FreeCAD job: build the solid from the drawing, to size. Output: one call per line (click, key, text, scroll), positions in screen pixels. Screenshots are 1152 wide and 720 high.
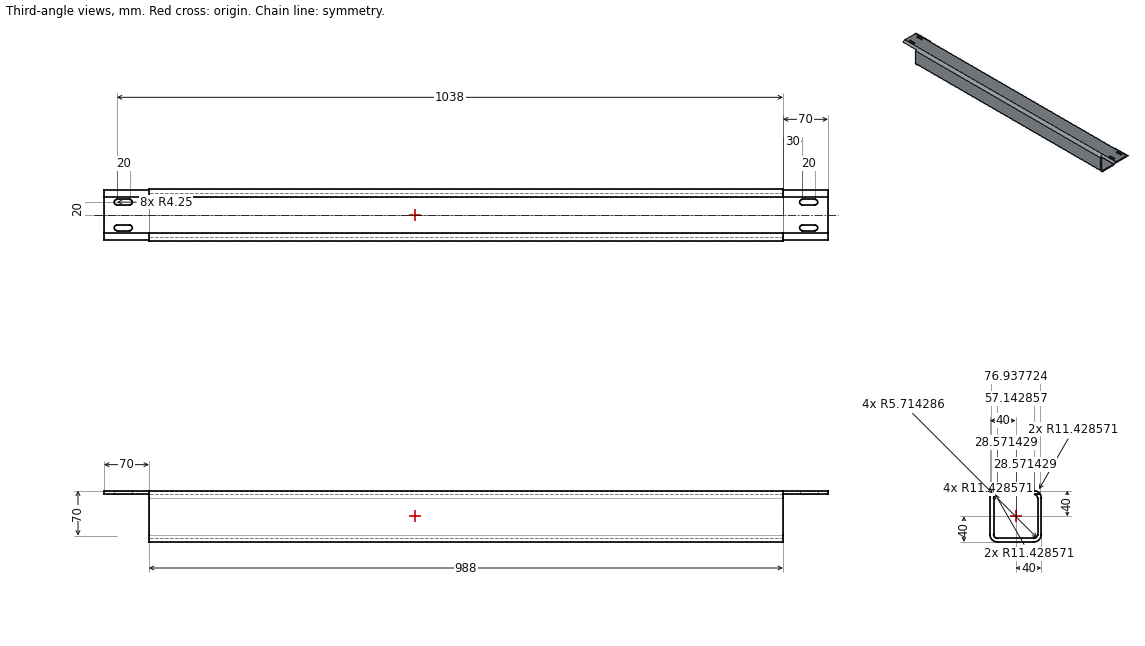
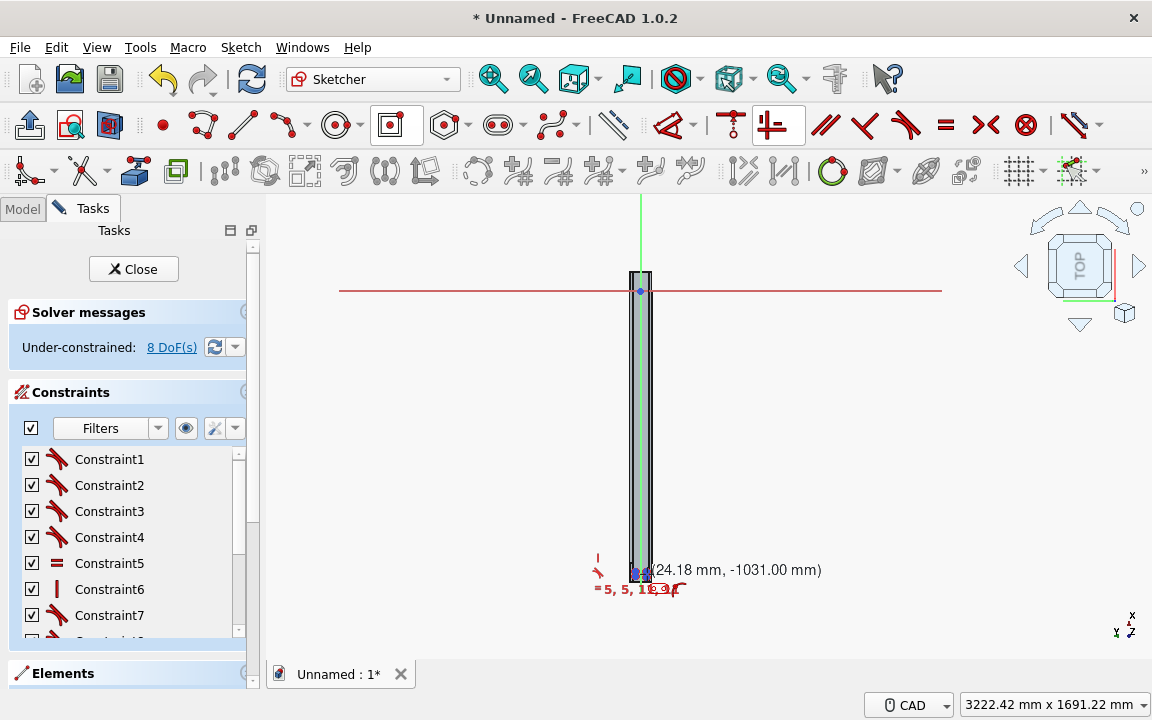
scroll(635, 283, up, 15)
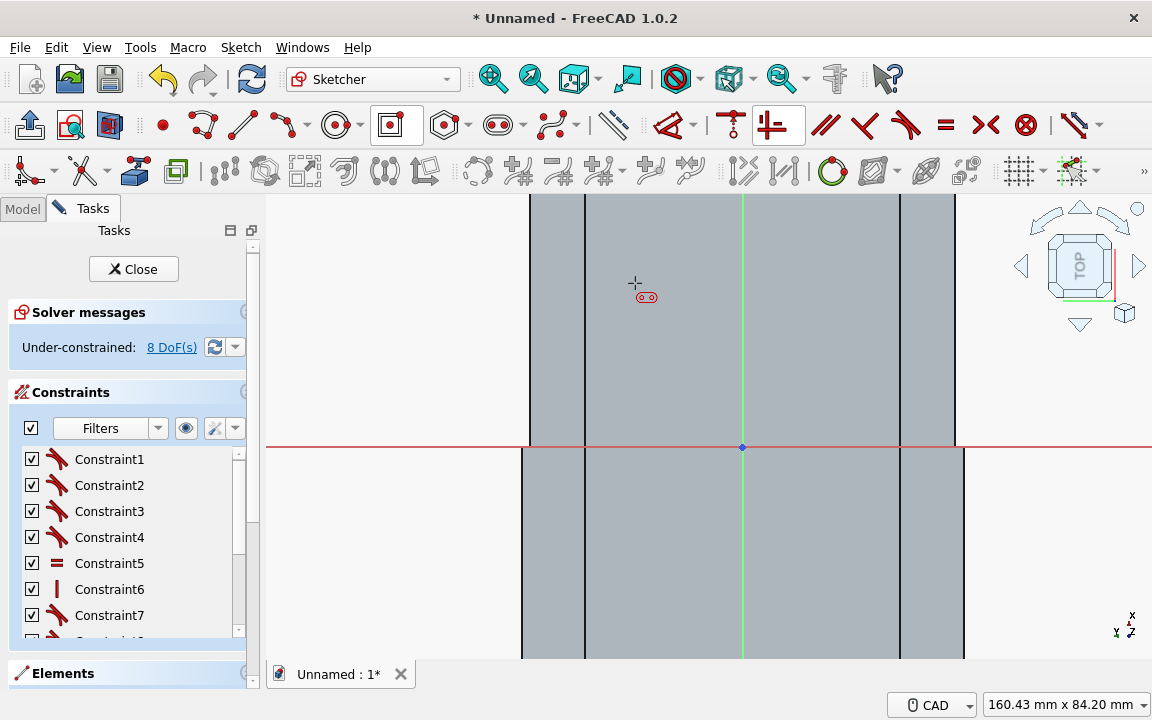
scroll(635, 282, down, 15)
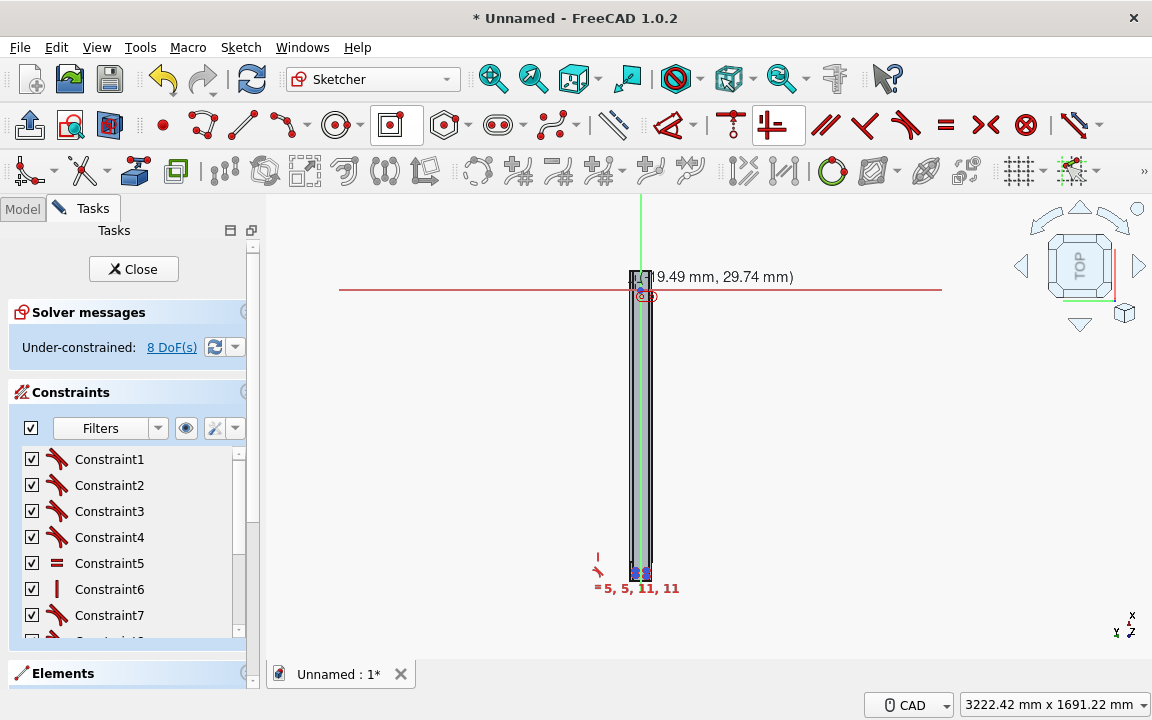
scroll(635, 282, up, 6)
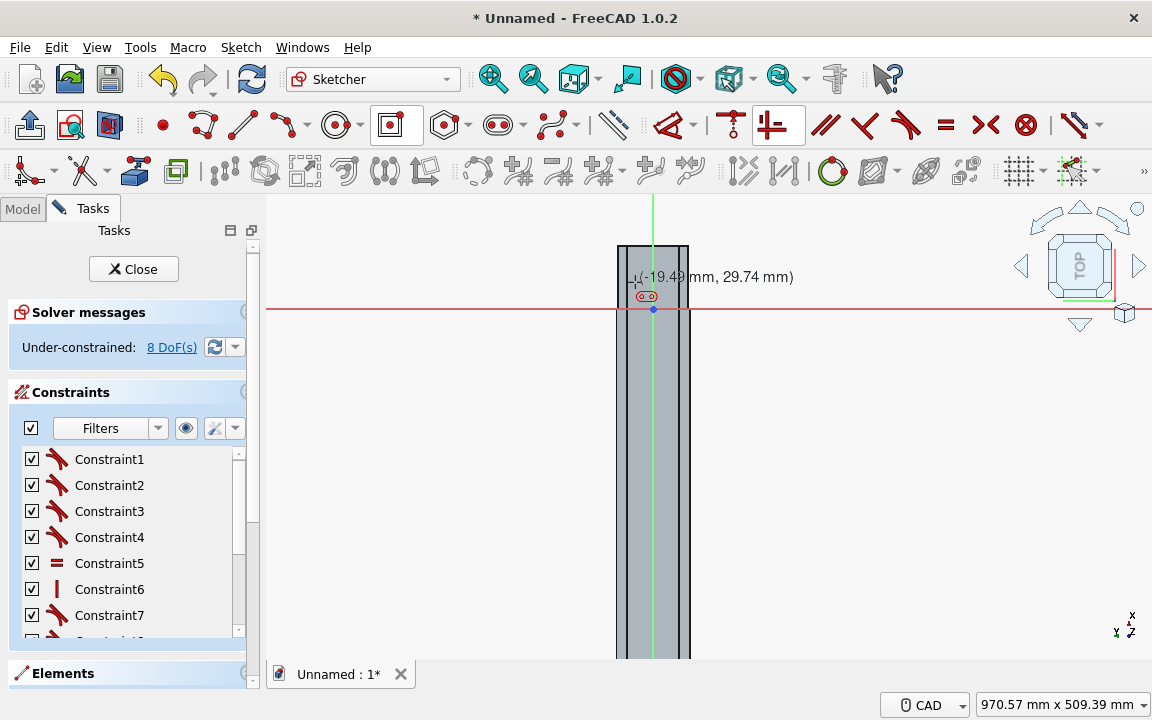
click(635, 282)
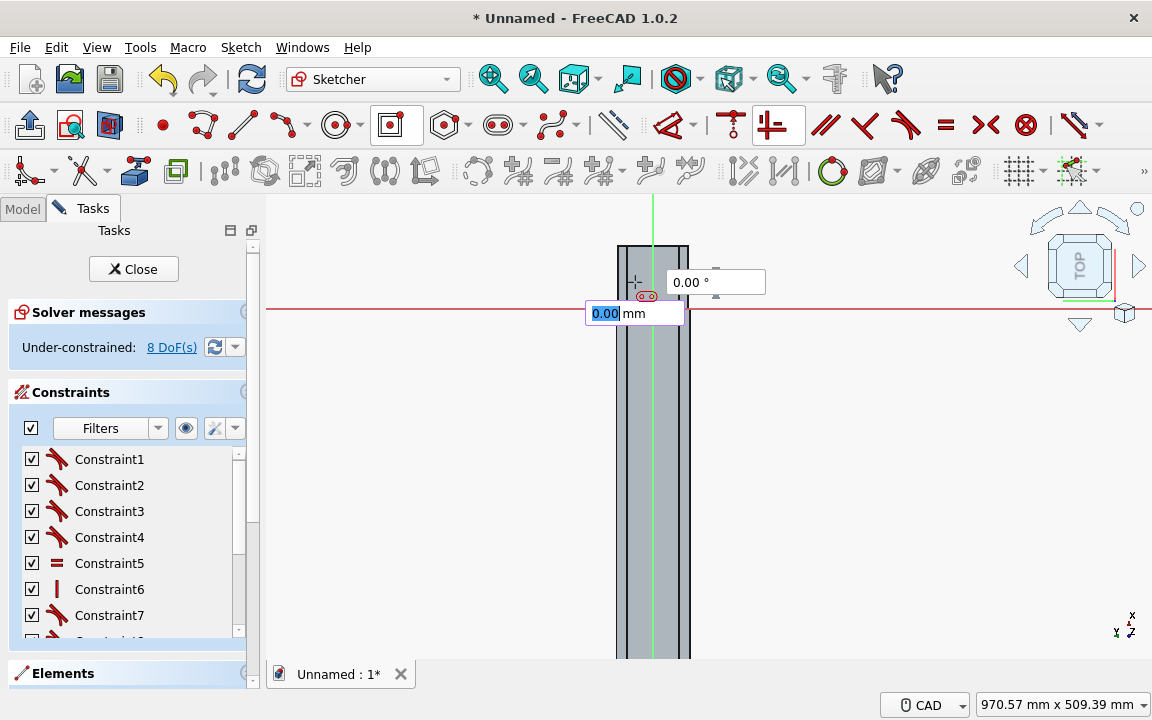
click(635, 264)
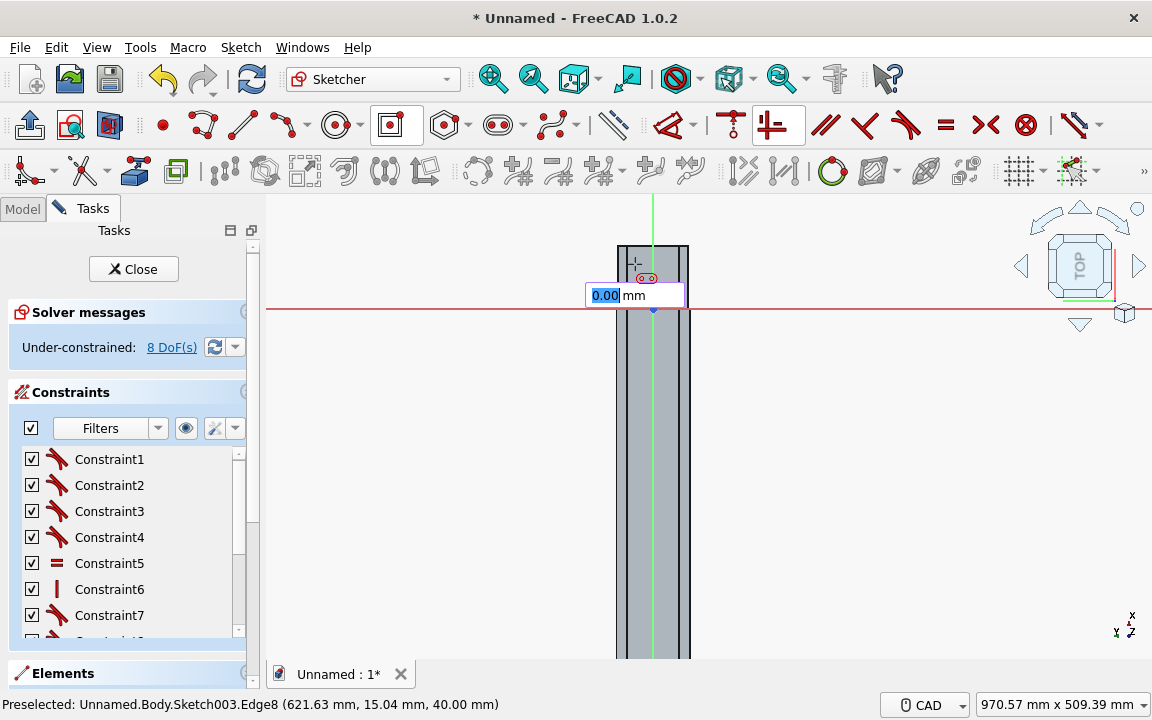
scroll(631, 273, up, 8)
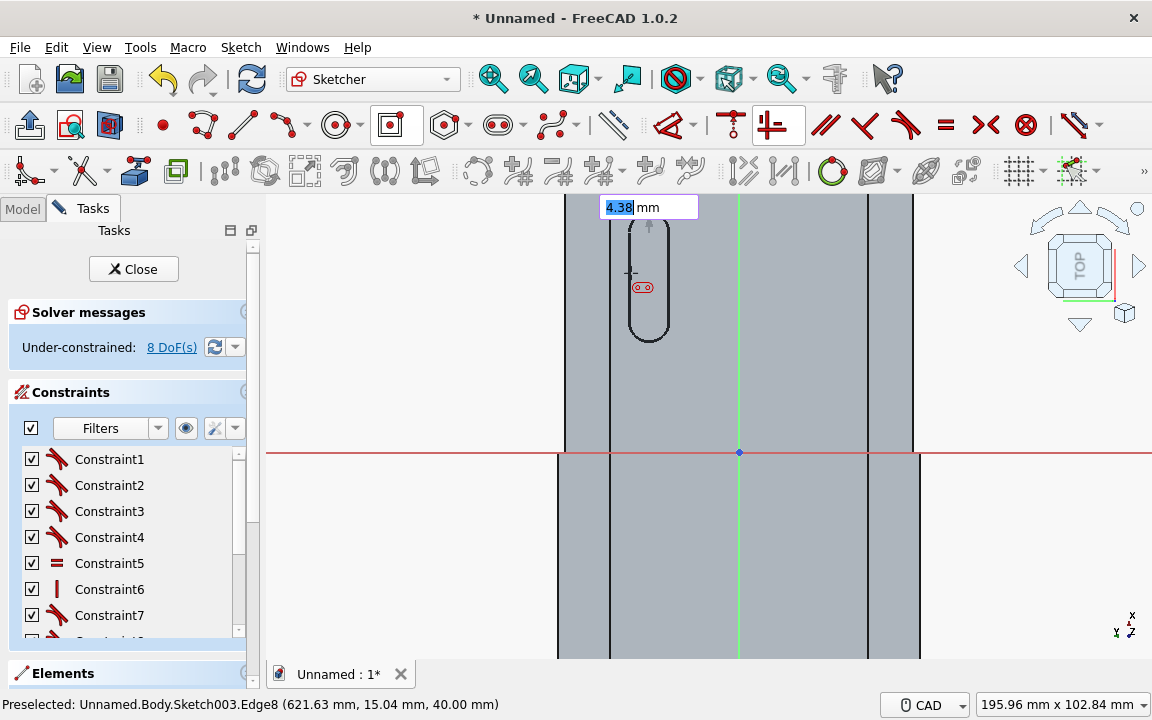
click(629, 272)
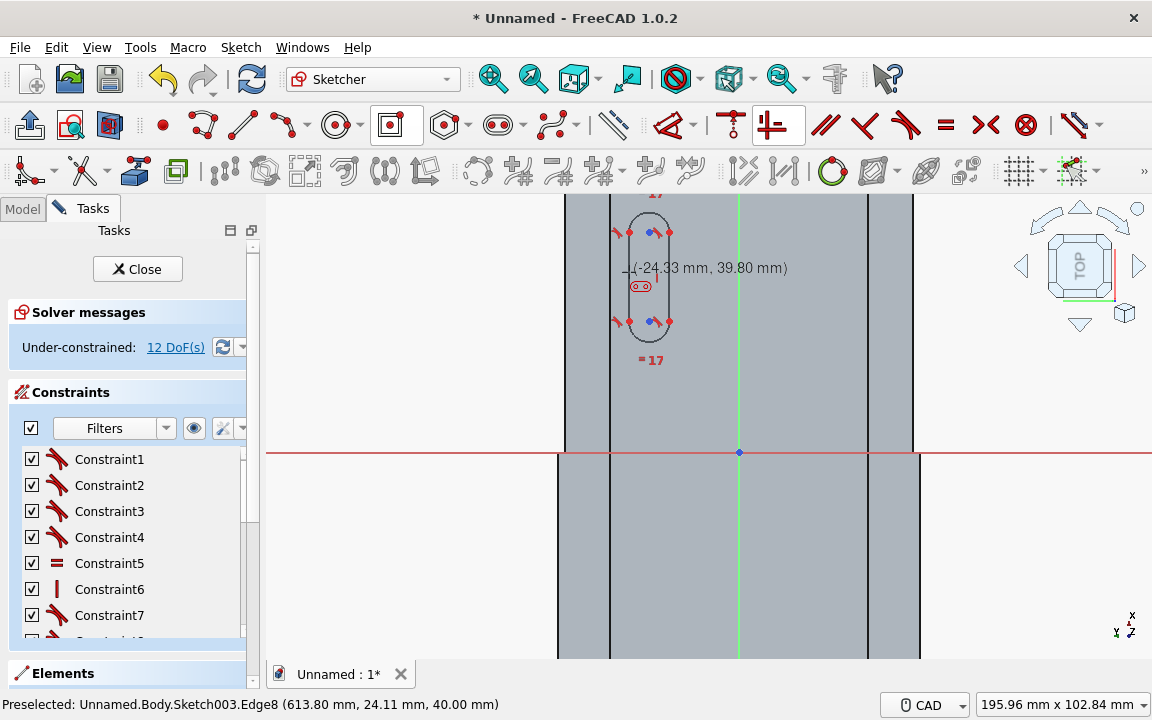
scroll(634, 280, down, 14)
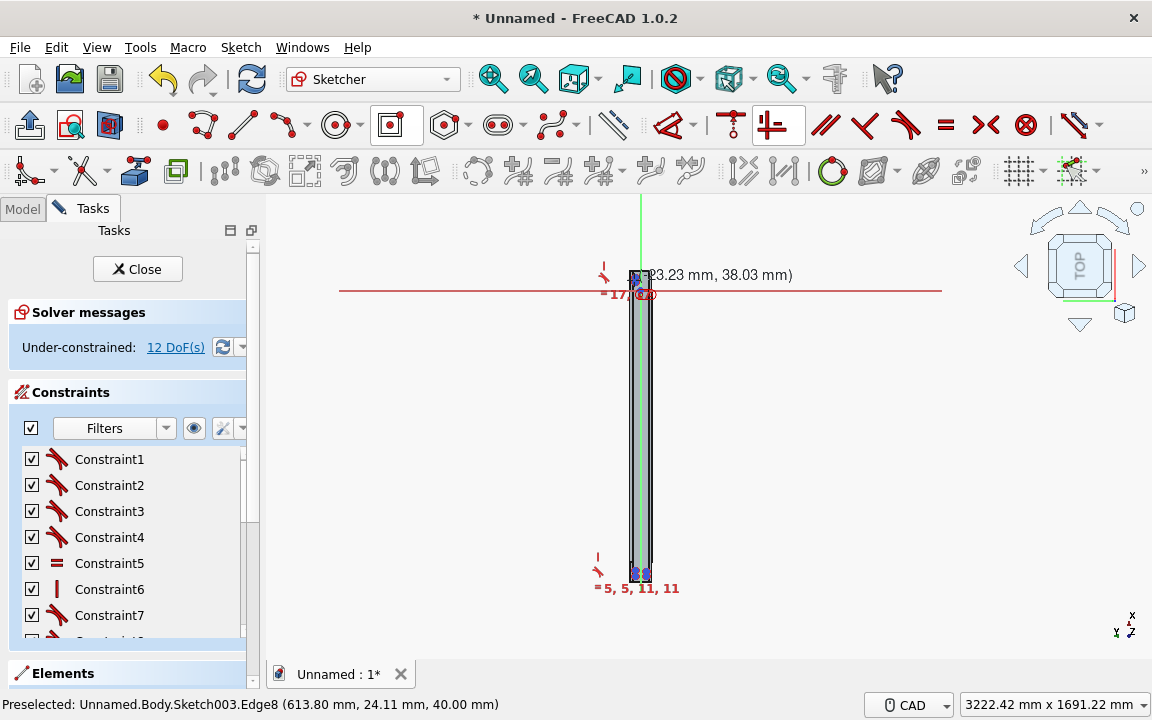
scroll(646, 282, up, 6)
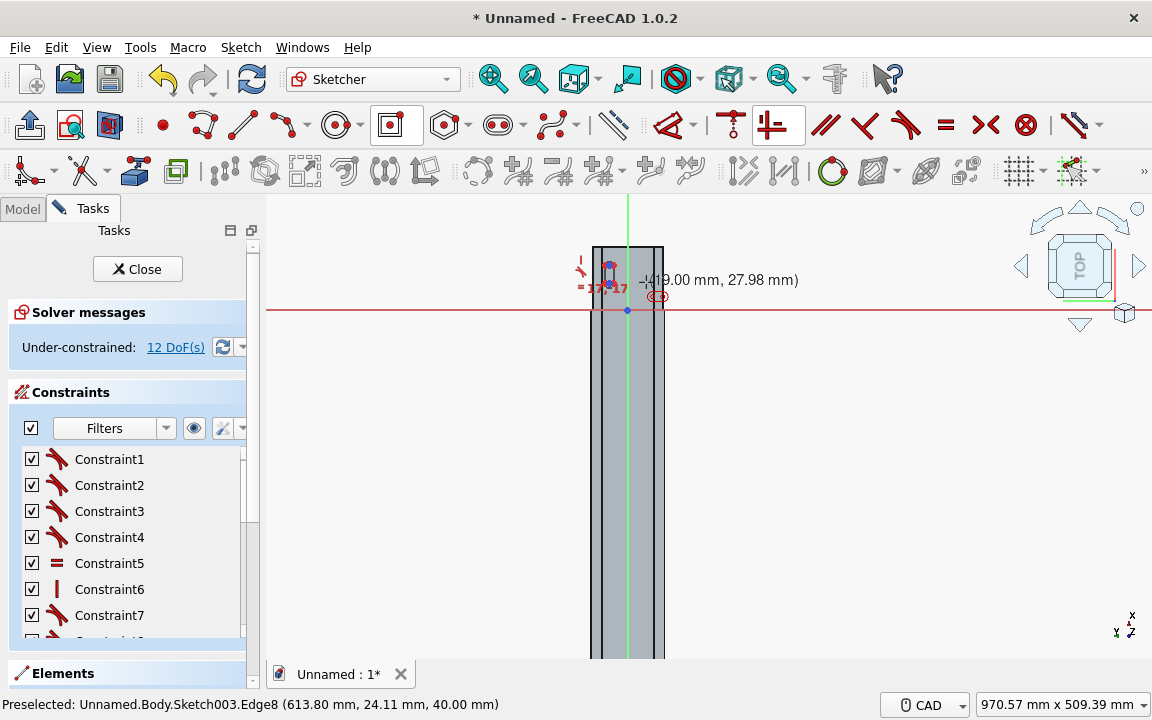
click(646, 283)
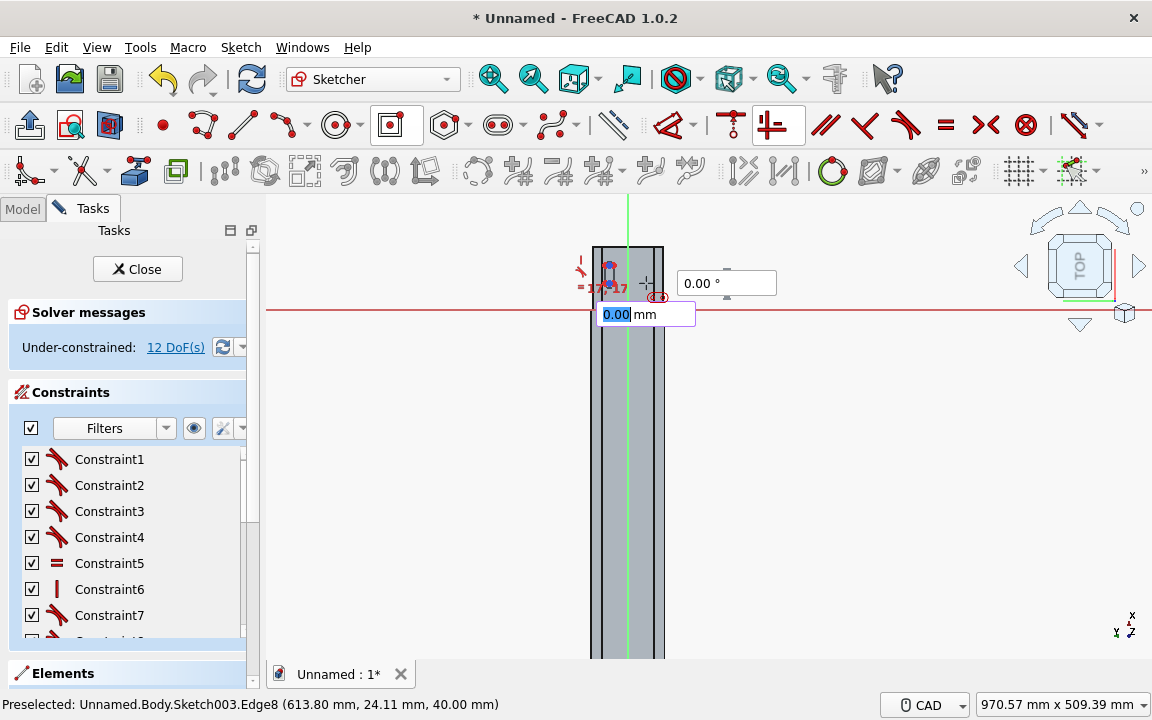
click(646, 265)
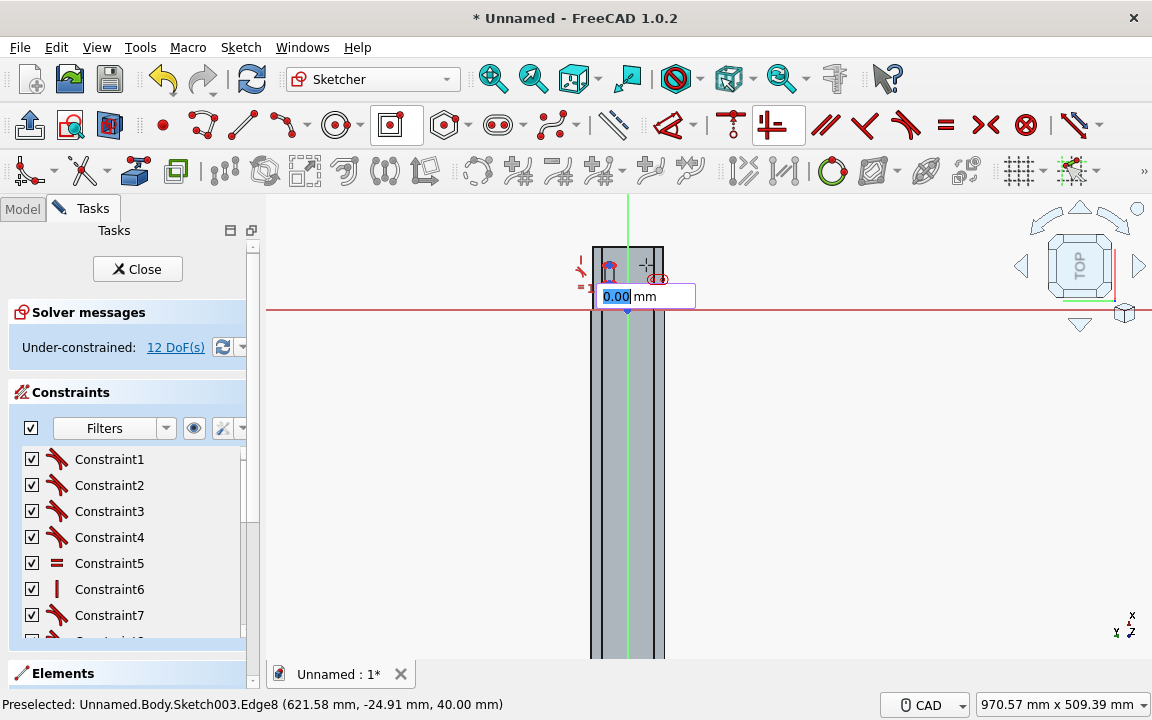
scroll(650, 274, up, 8)